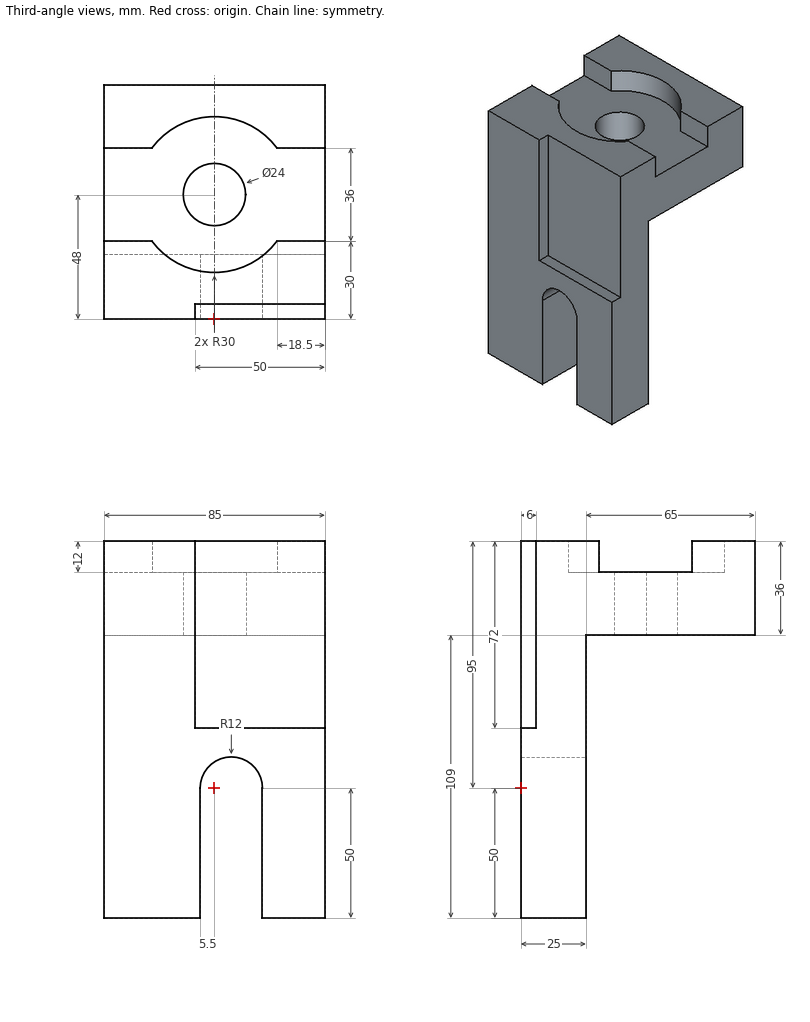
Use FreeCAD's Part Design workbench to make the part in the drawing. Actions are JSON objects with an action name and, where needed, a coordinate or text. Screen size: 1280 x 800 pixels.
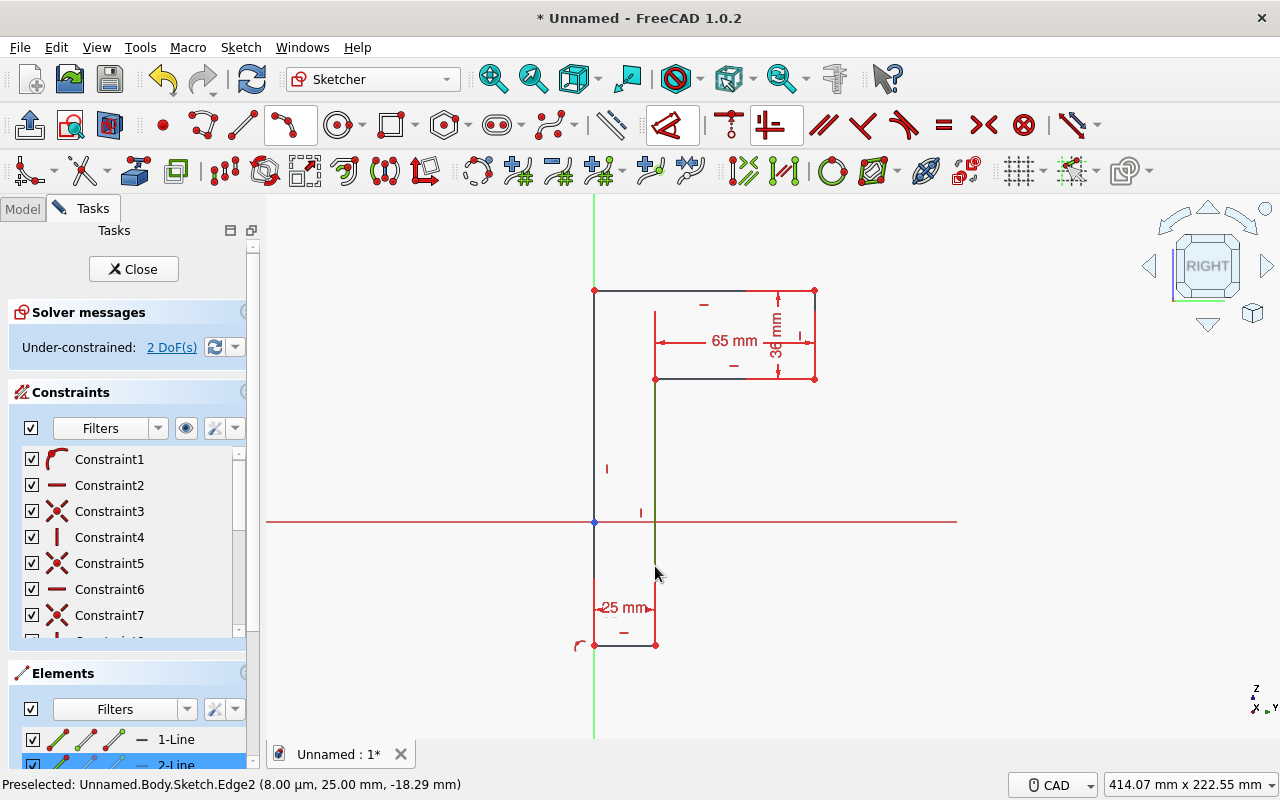
{"action": "key", "text": "i"}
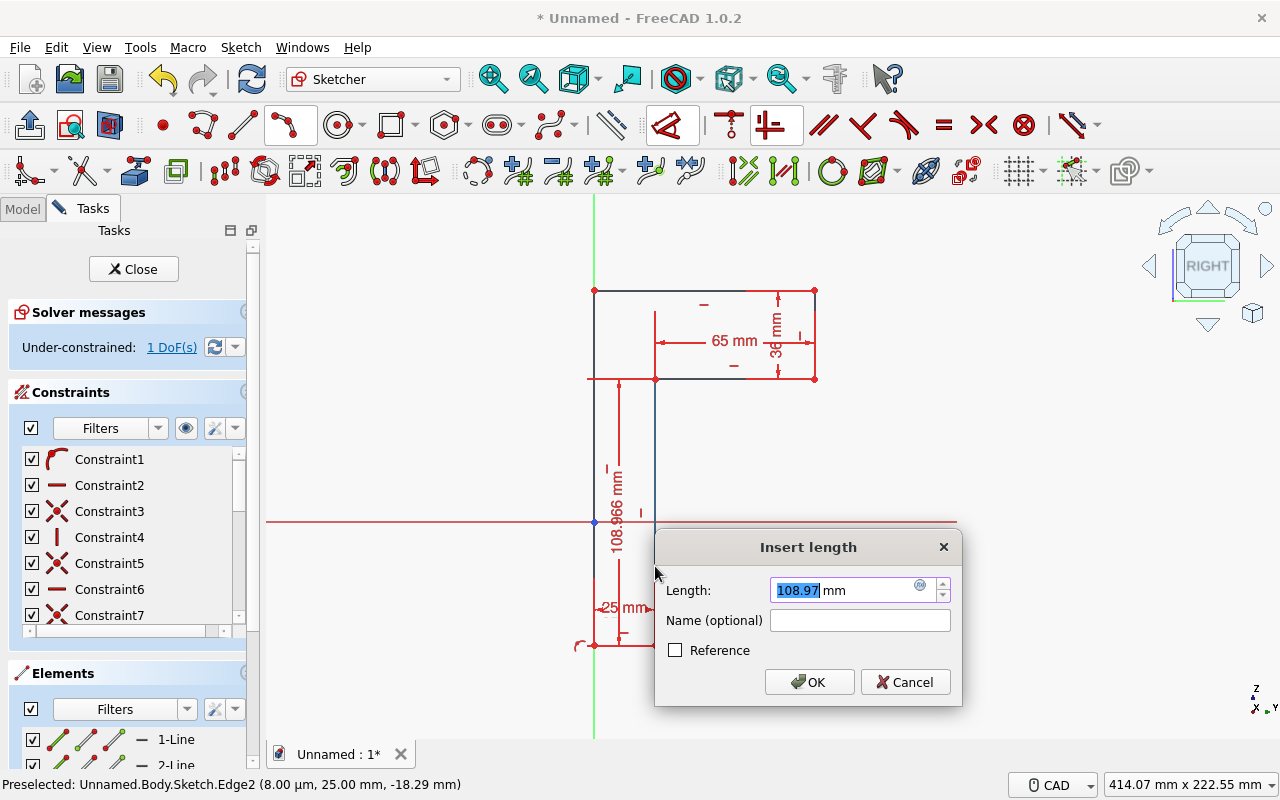
{"action": "type", "text": "109"}
{"action": "key", "text": "Return"}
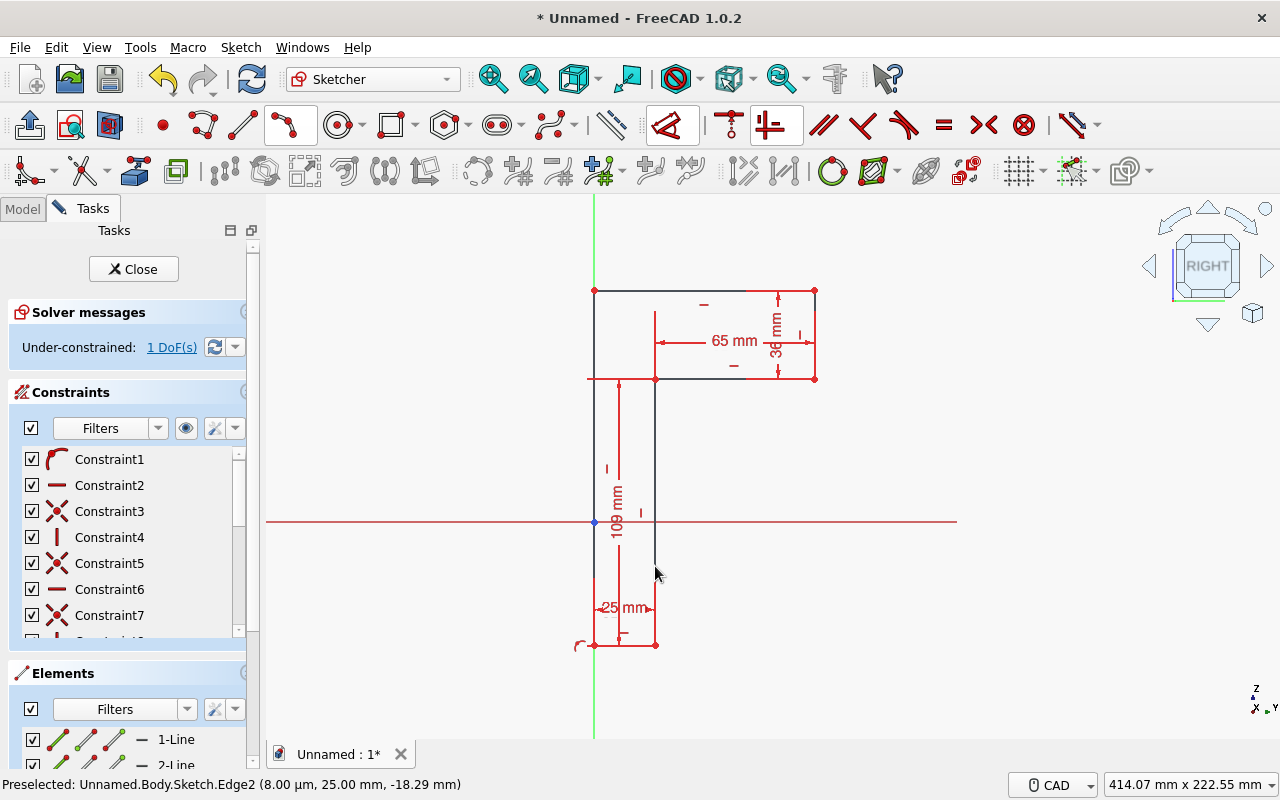
{"action": "left_click", "coordinate": [594, 646]}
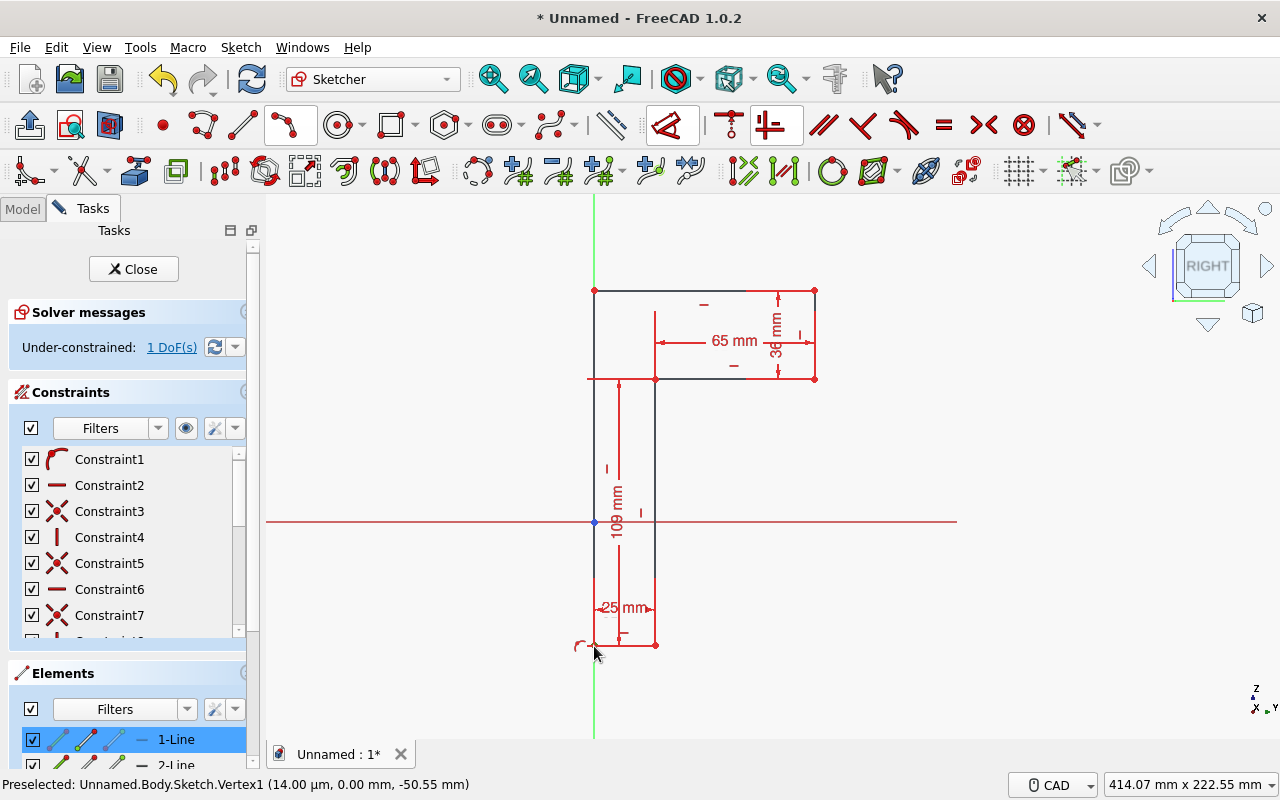
{"action": "key", "text": "i"}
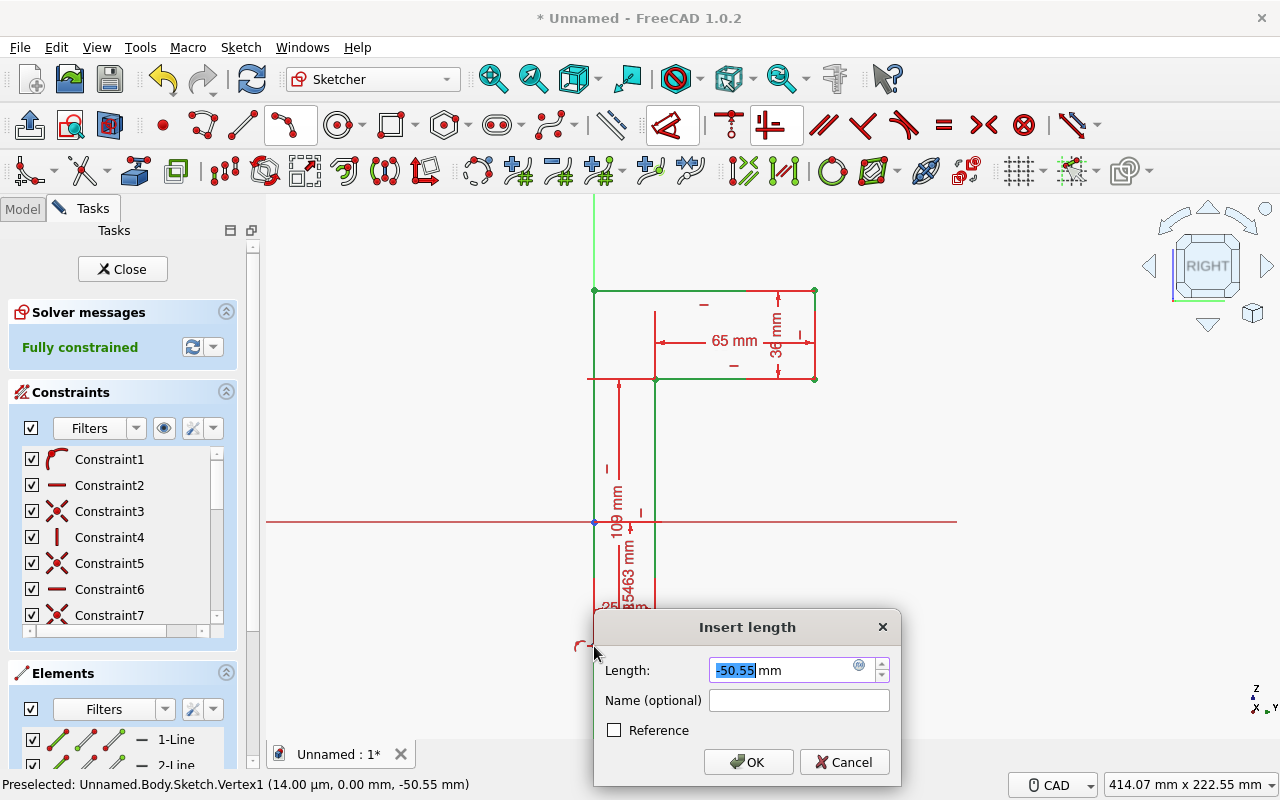
{"action": "type", "text": "-50"}
{"action": "key", "text": "Return"}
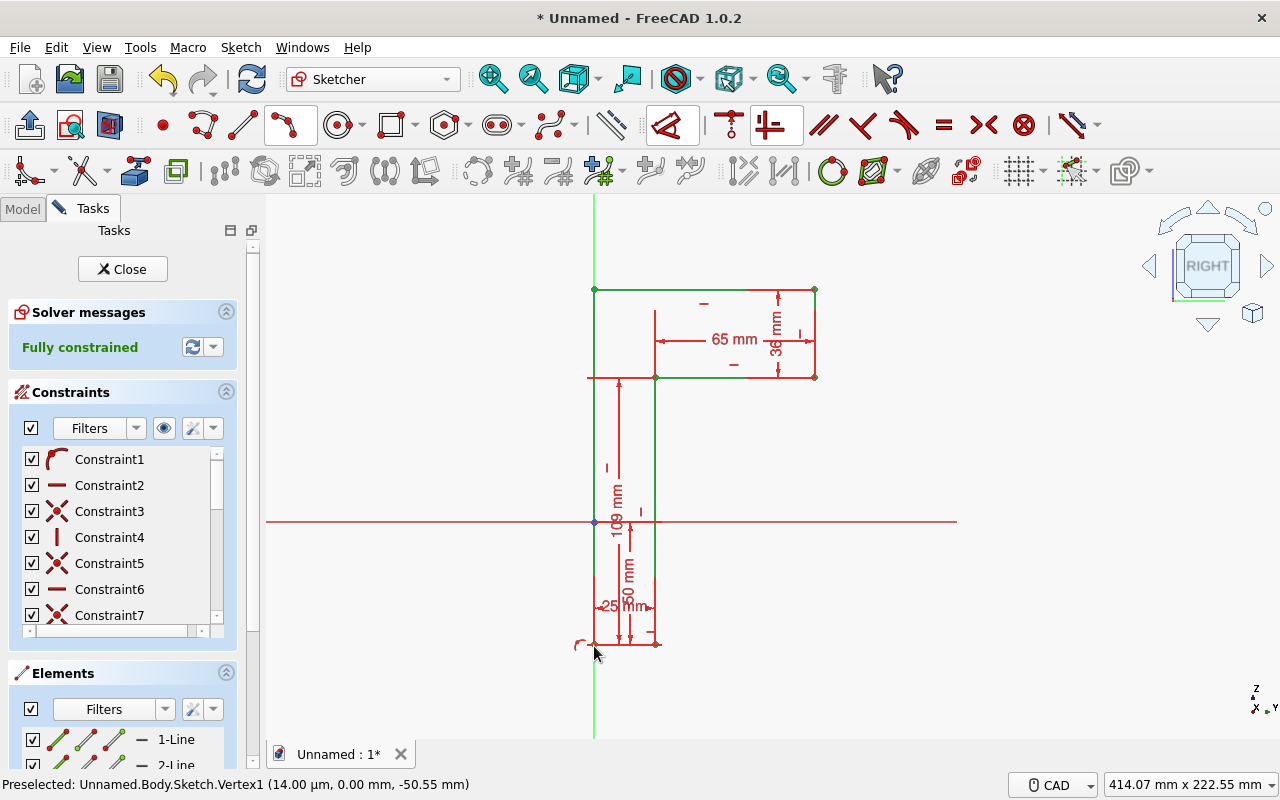
{"action": "left_click", "coordinate": [123, 269]}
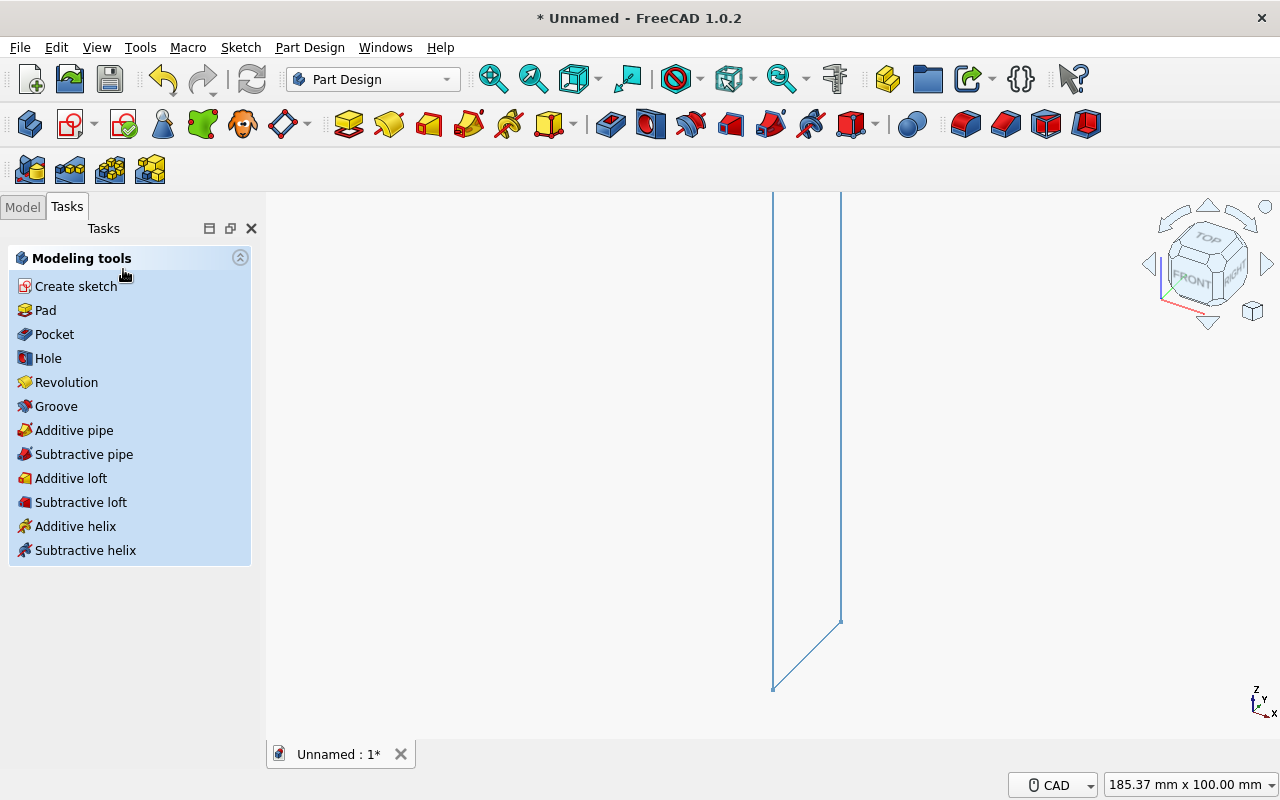
{"action": "left_click", "coordinate": [350, 124]}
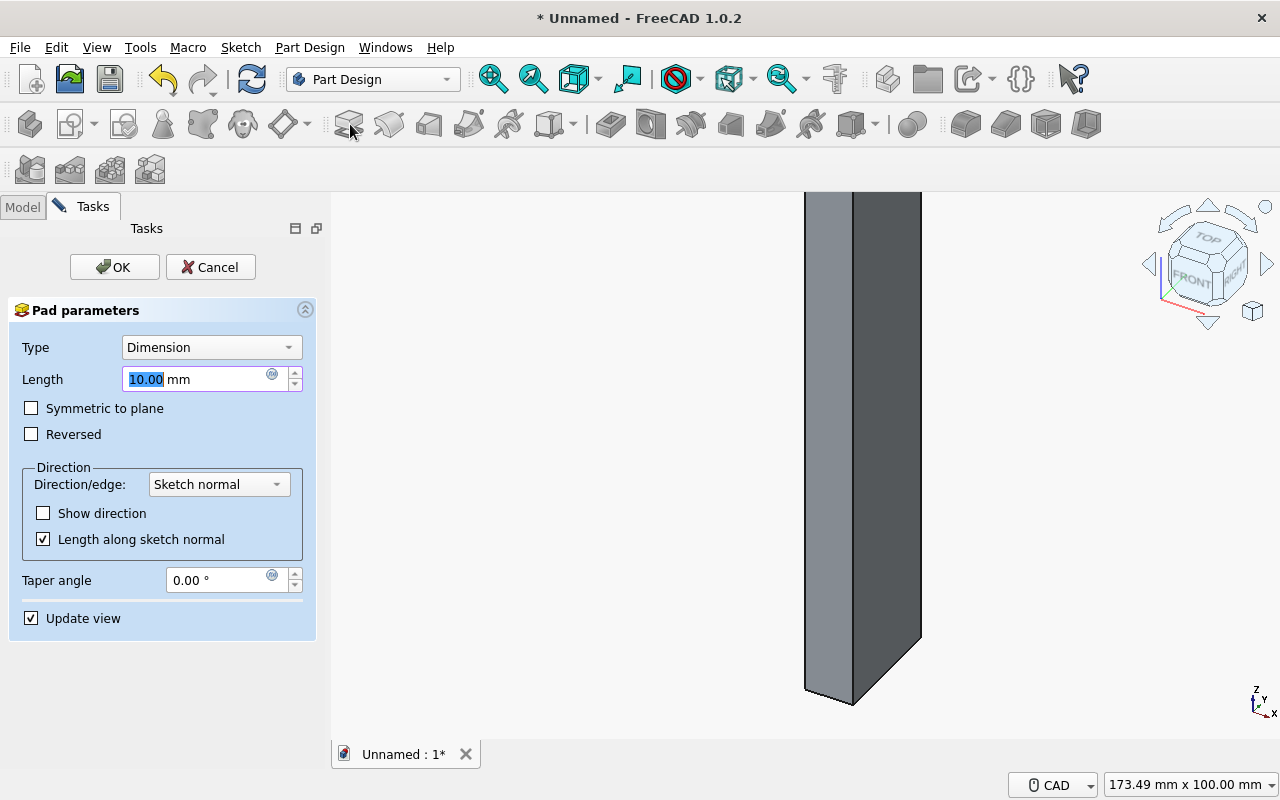
{"action": "type", "text": "85"}
{"action": "key", "text": "Tab"}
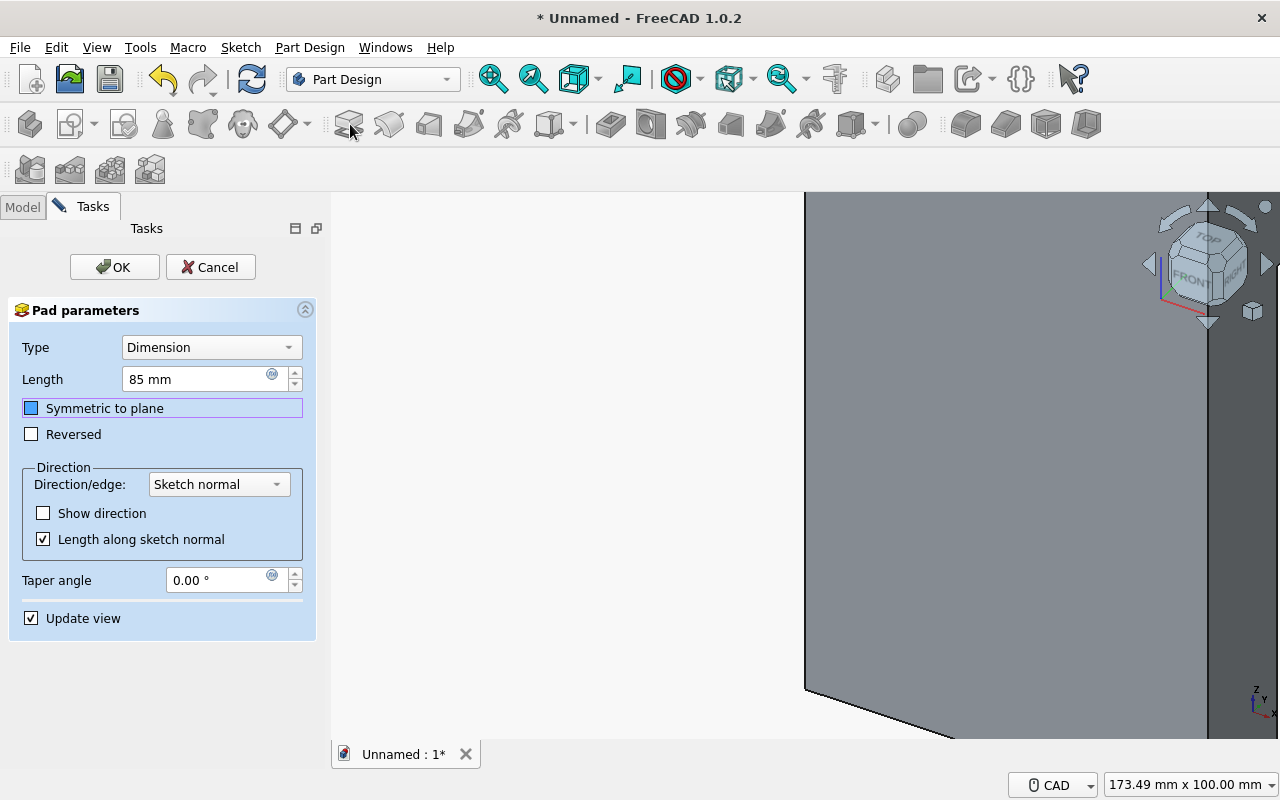
{"action": "left_click", "coordinate": [30, 408]}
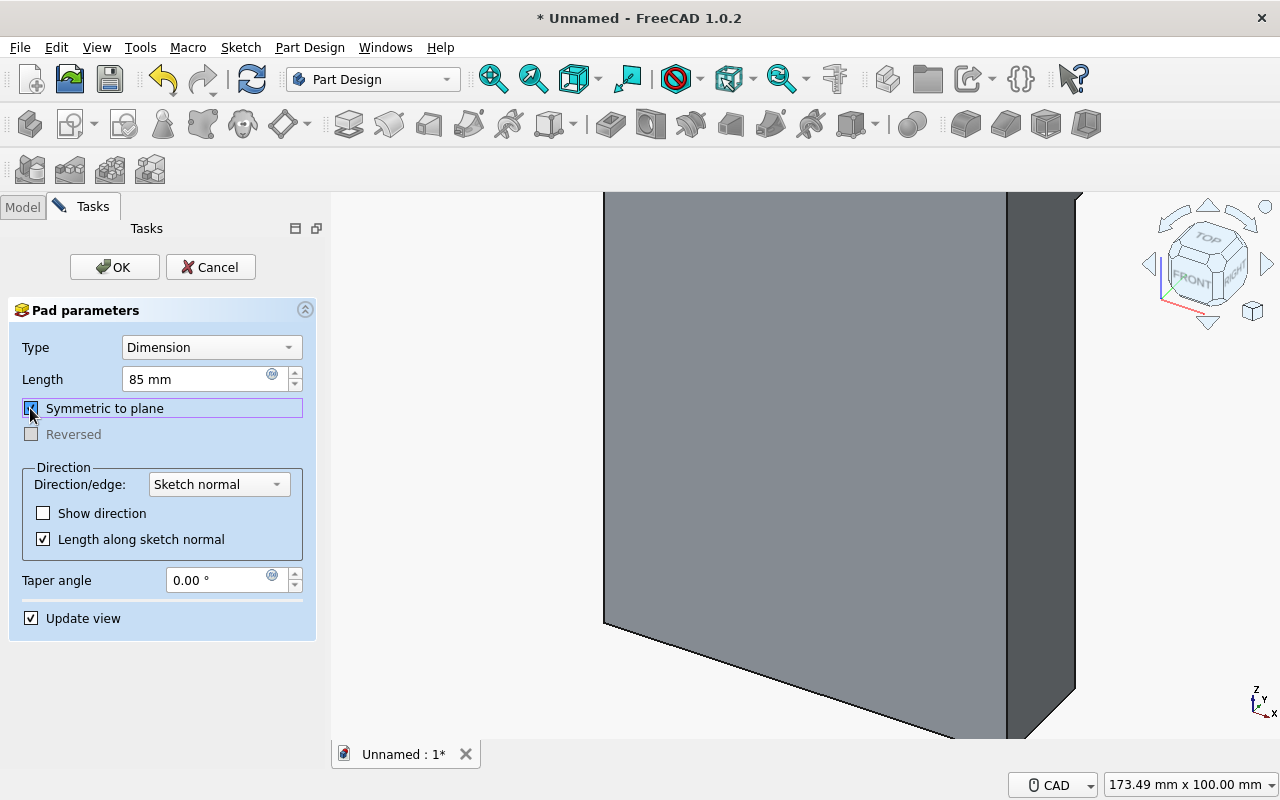
{"action": "left_click", "coordinate": [115, 267]}